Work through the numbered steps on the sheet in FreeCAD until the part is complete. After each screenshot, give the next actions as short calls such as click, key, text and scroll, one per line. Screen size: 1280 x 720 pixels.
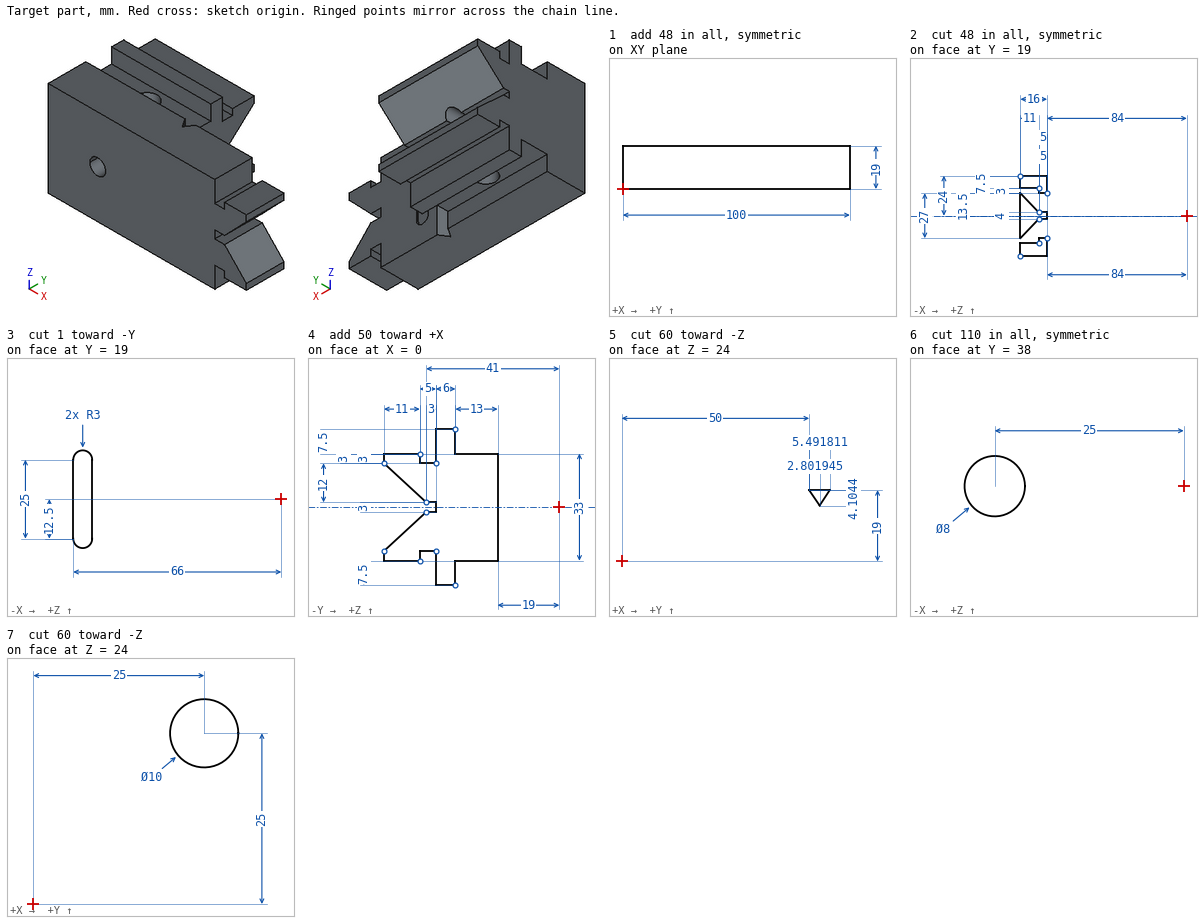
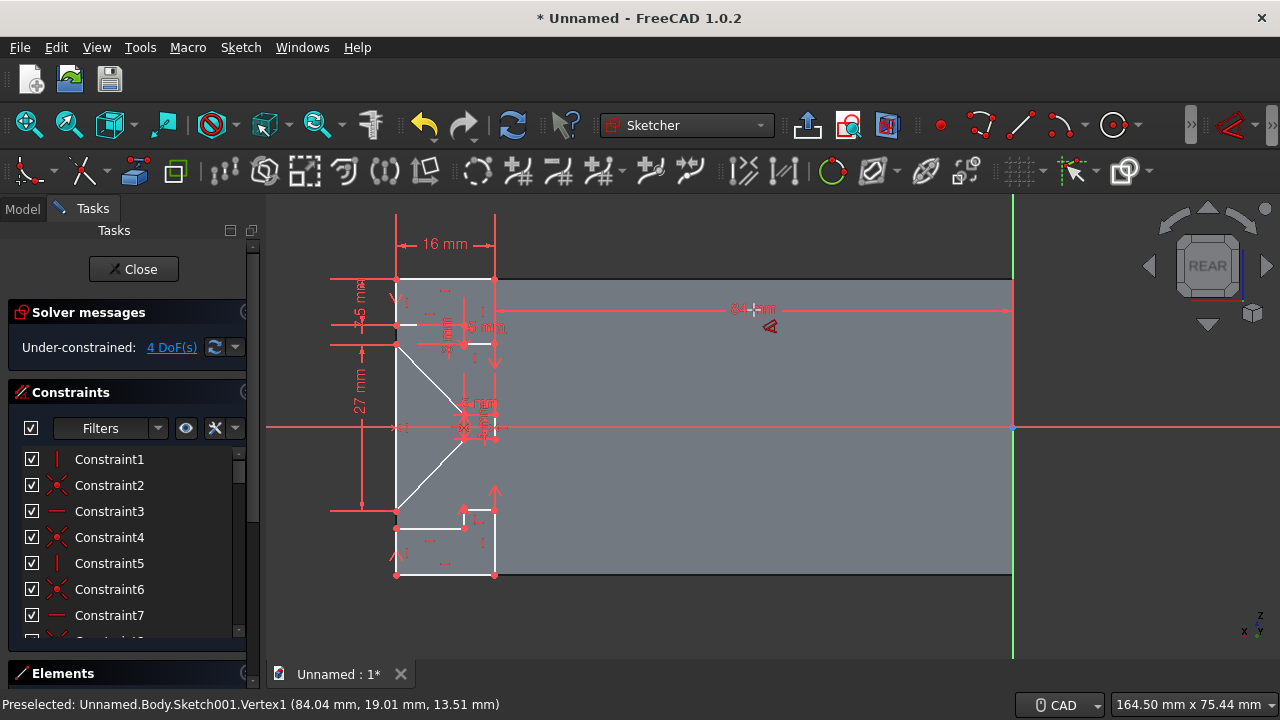
click(495, 279)
click(1047, 353)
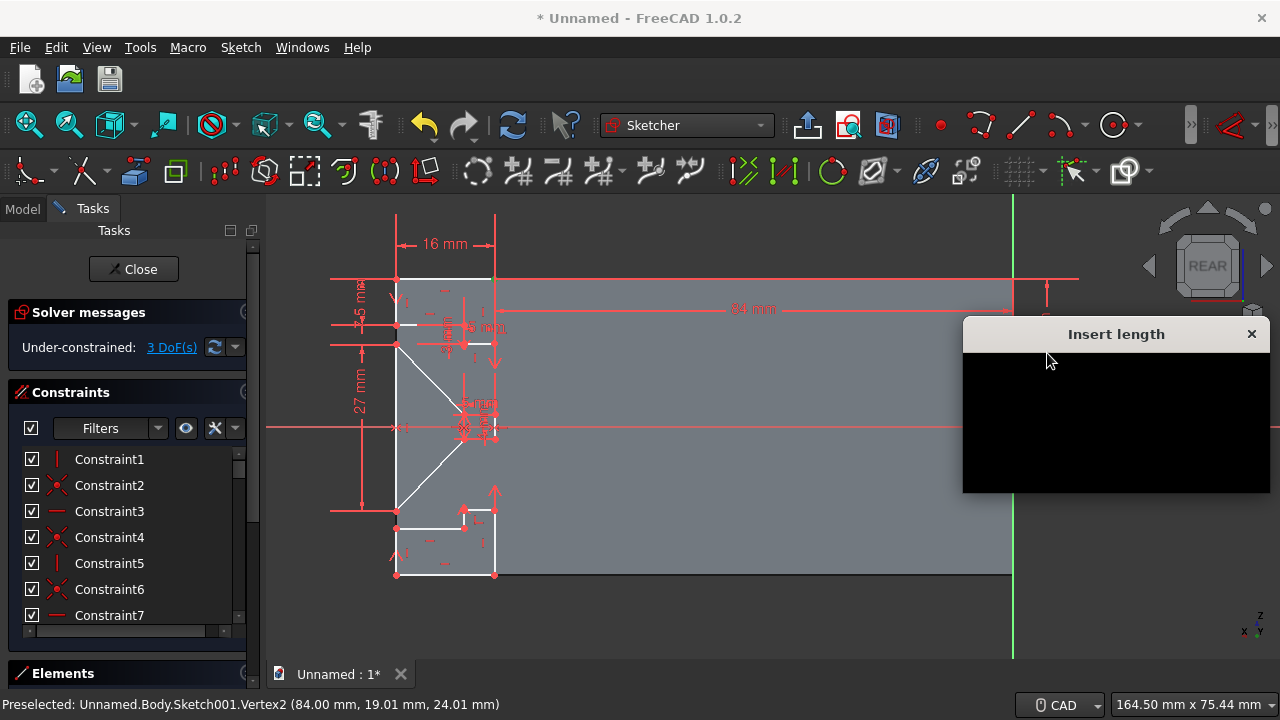
text(24)
key(Return)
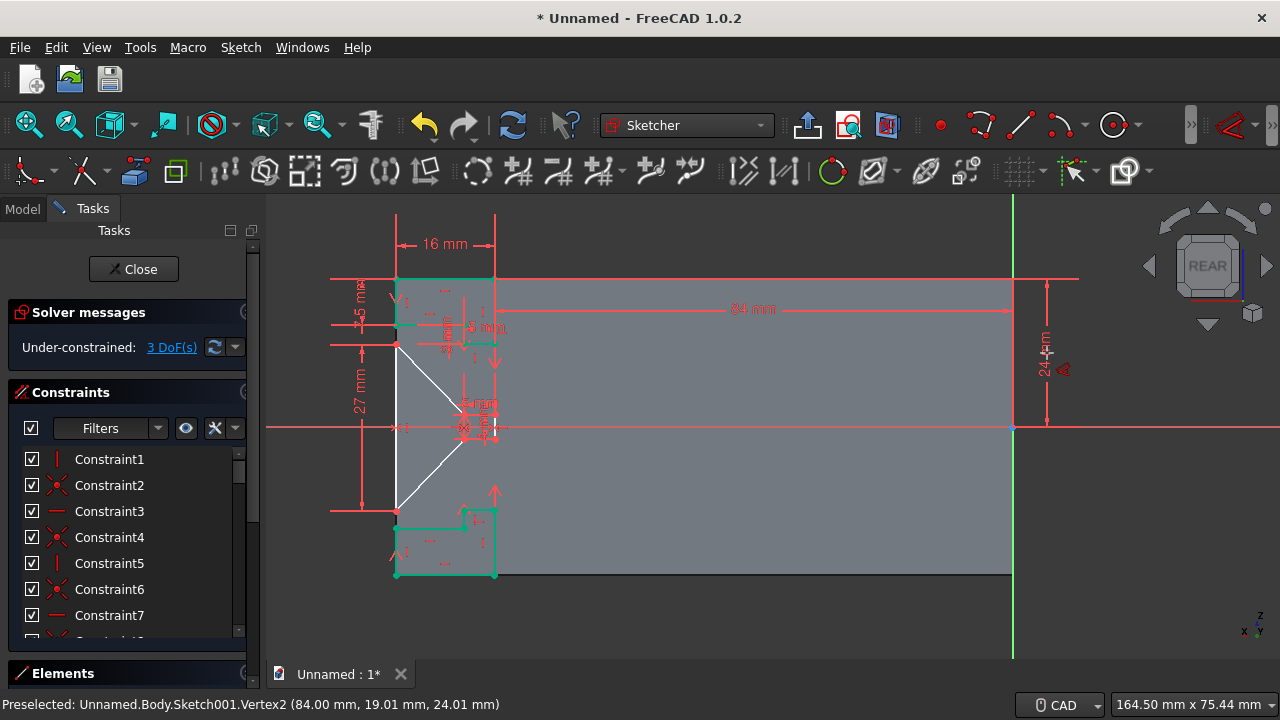
click(495, 439)
click(754, 473)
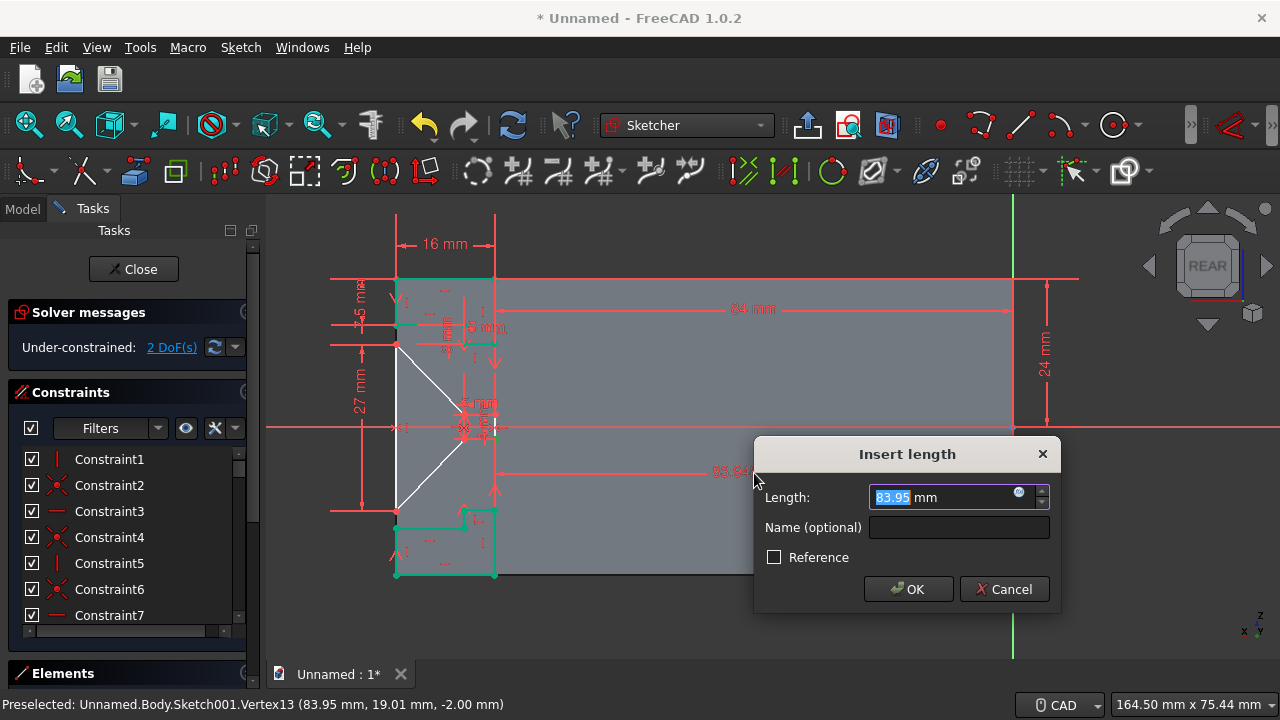
text(84)
key(Return)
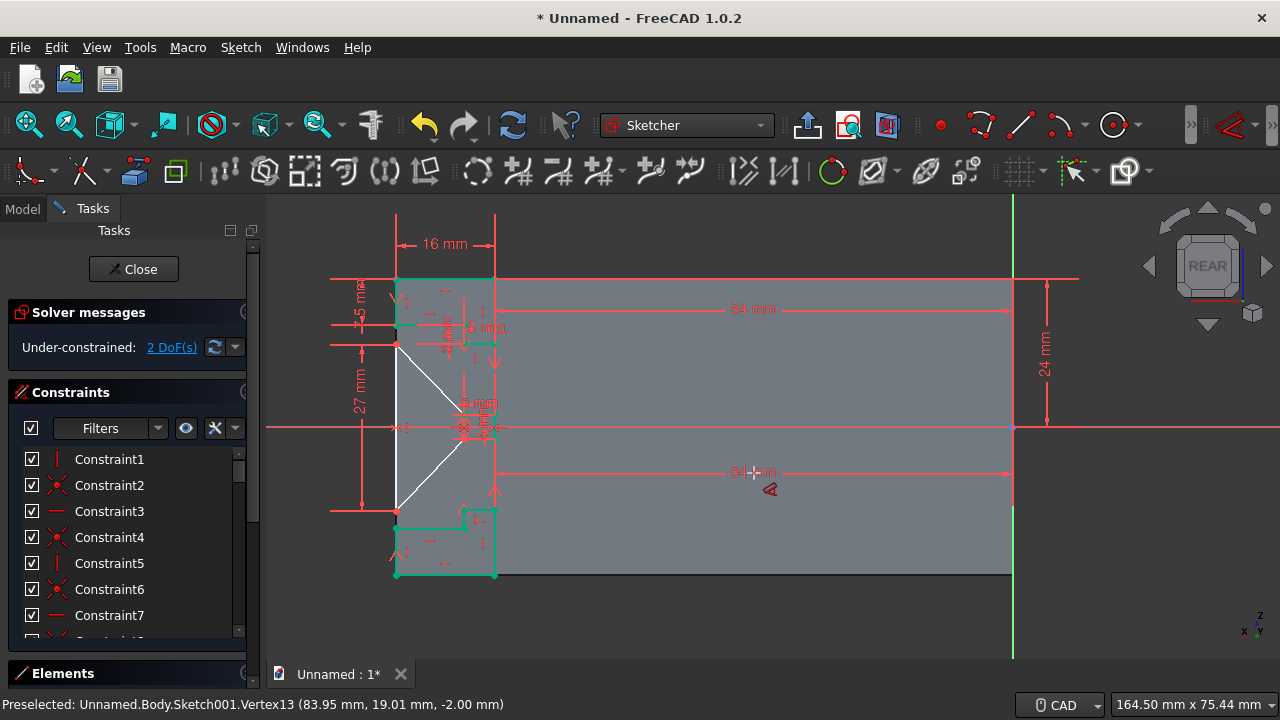
click(444, 394)
click(430, 449)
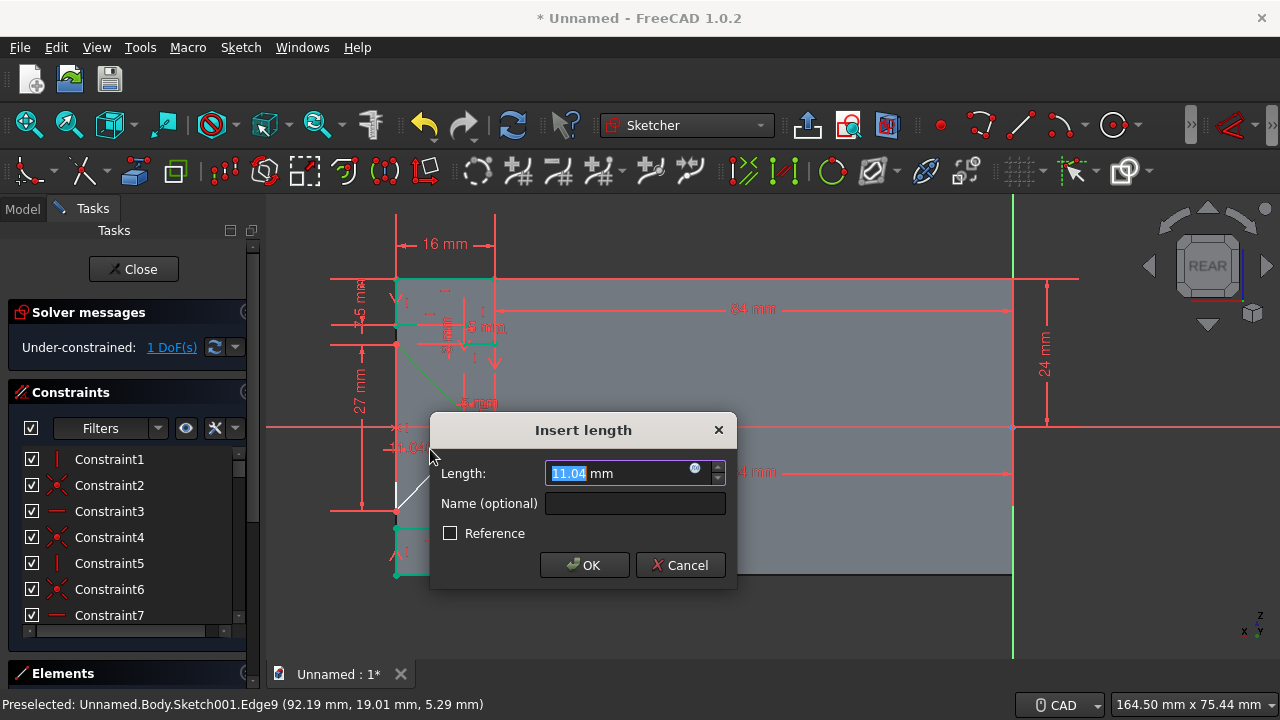
text(11)
key(Return)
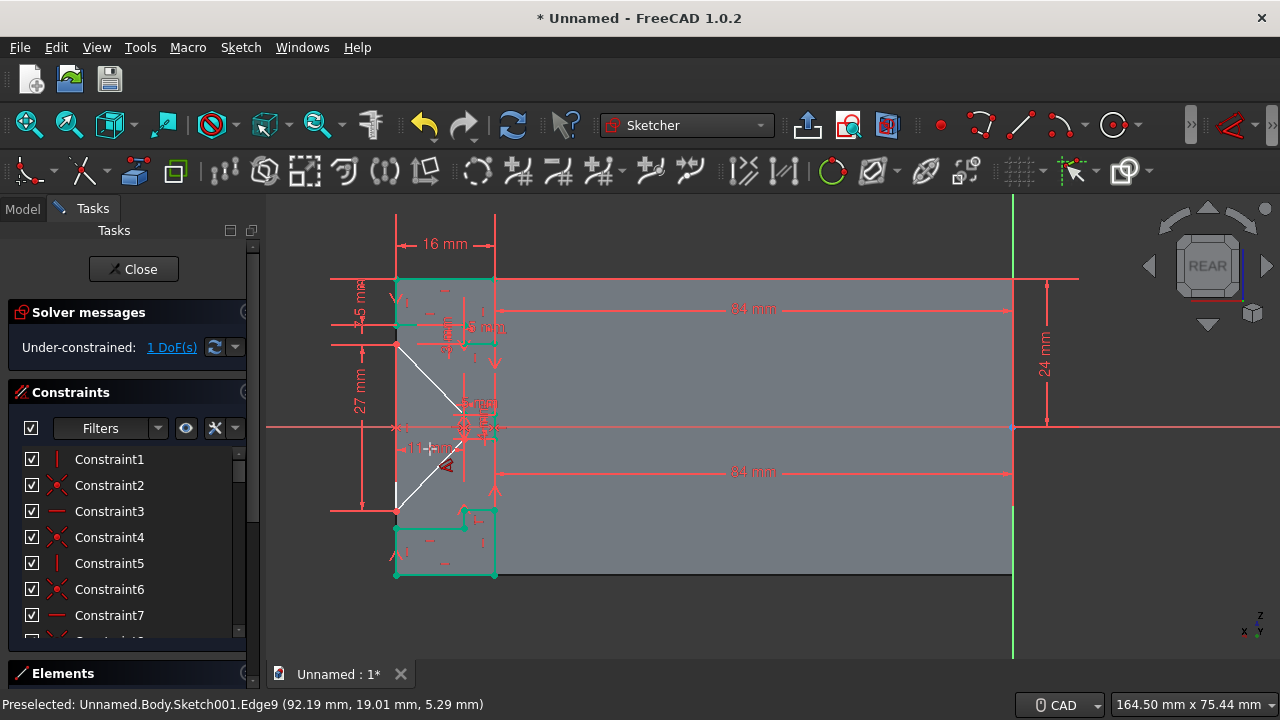
click(396, 345)
click(1047, 386)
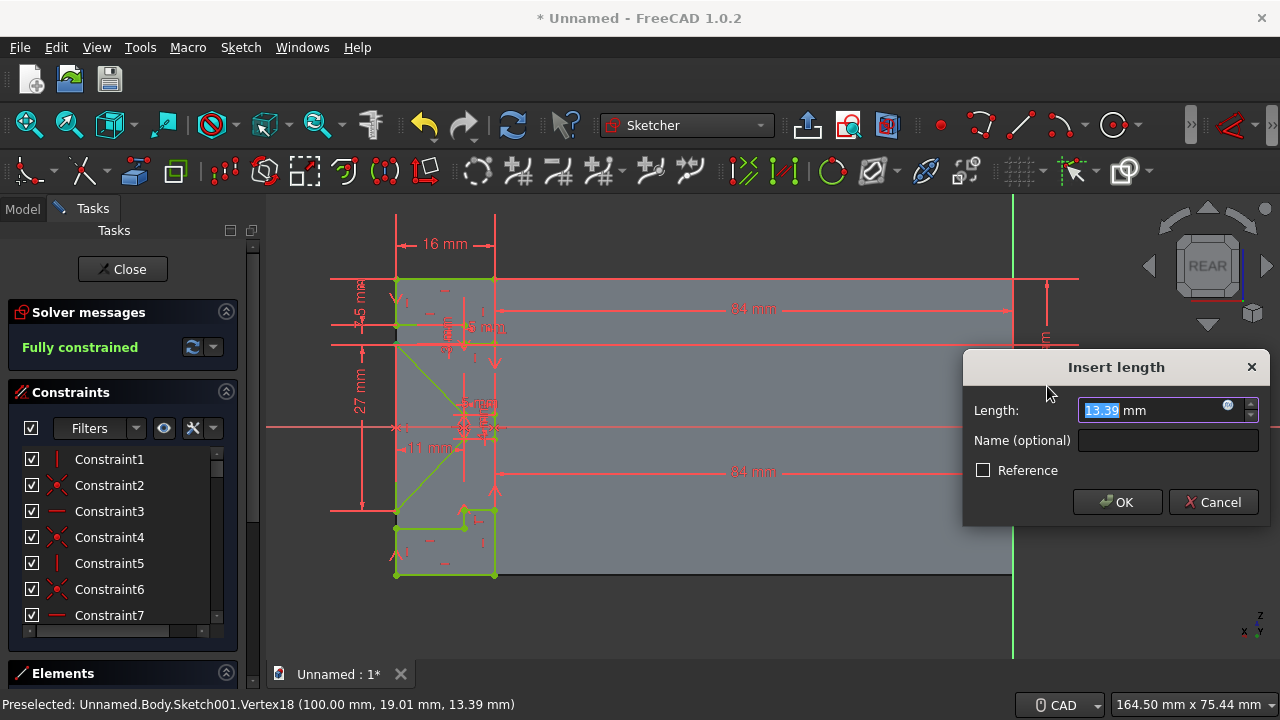
text(13.5)
key(Return)
key(Escape)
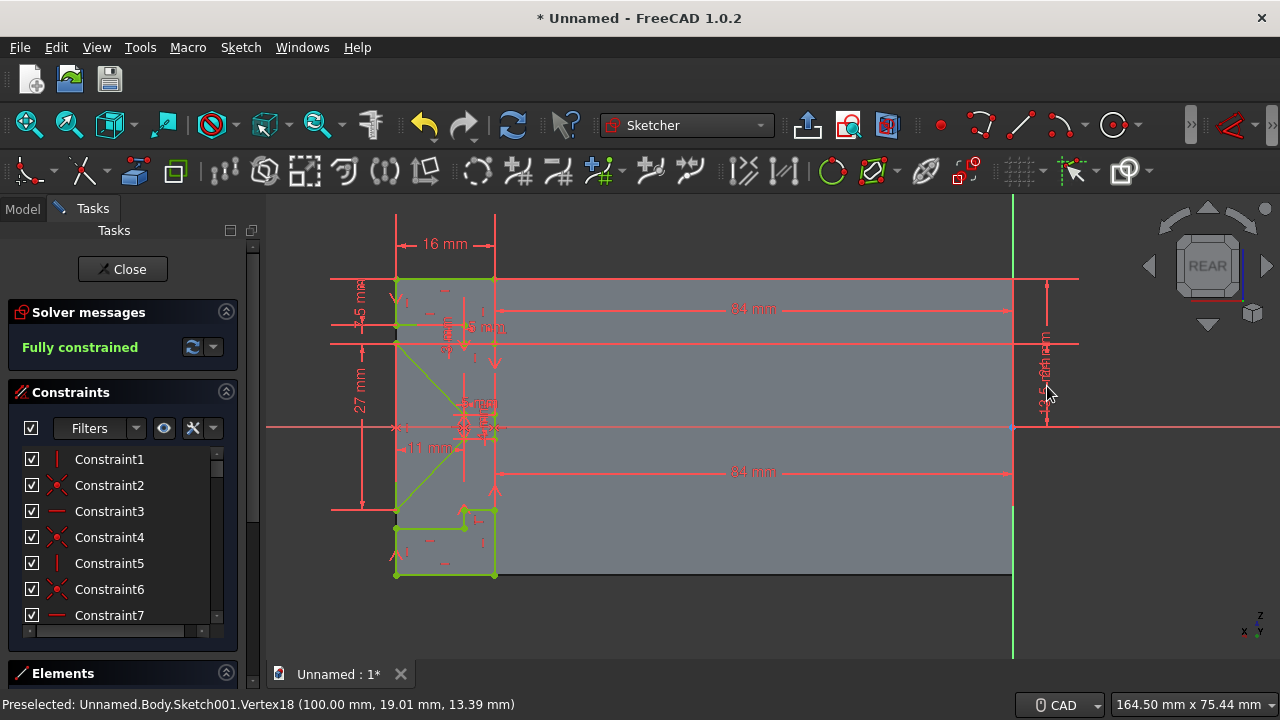
click(123, 269)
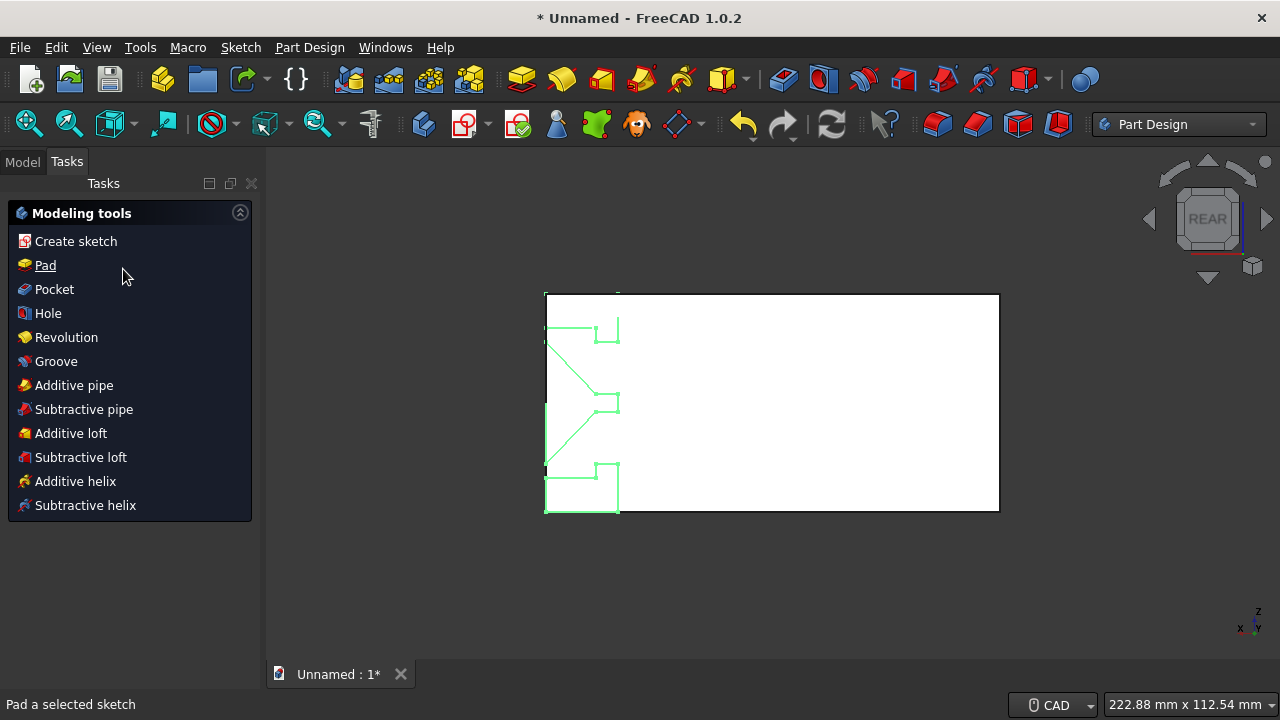
click(784, 80)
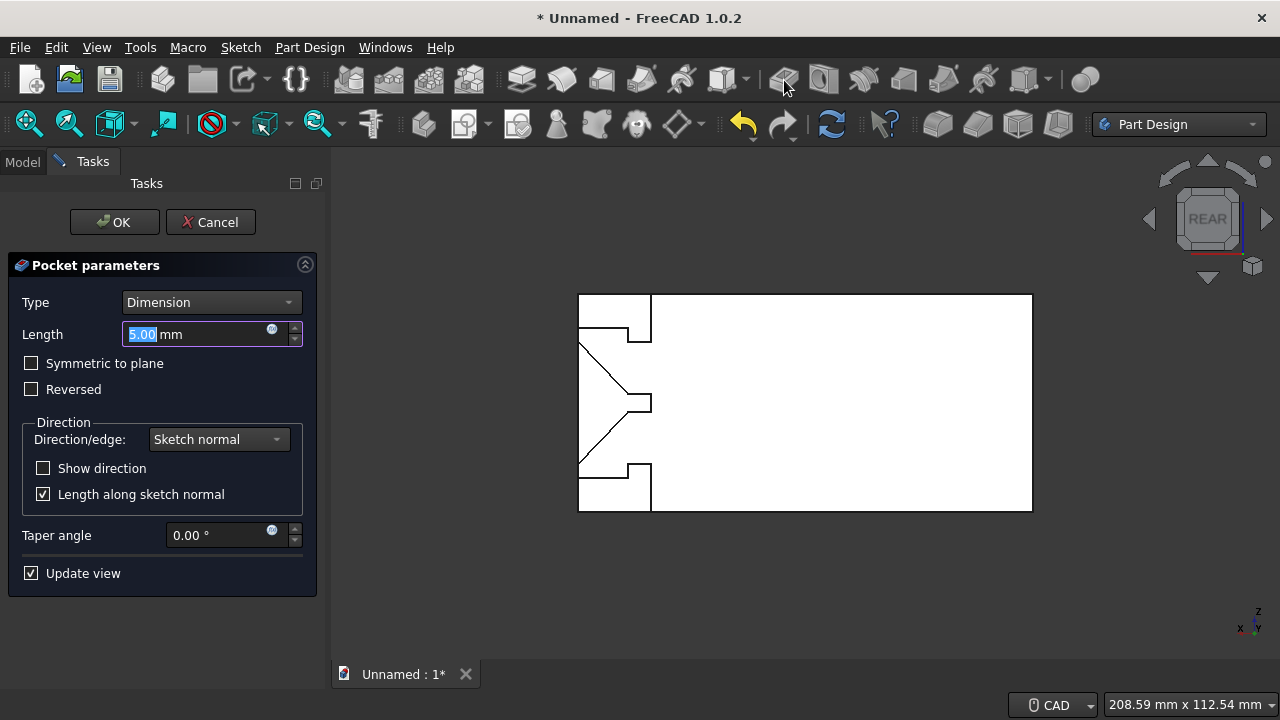
text(48)
key(Tab)